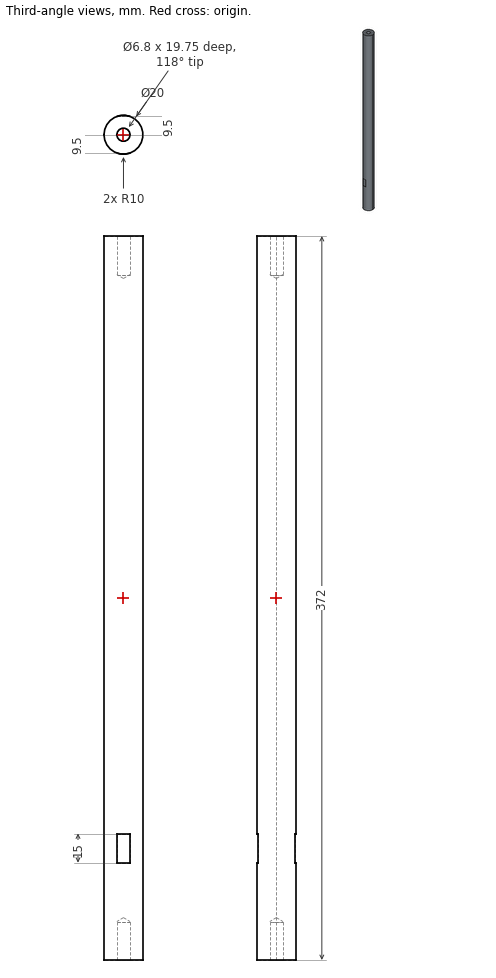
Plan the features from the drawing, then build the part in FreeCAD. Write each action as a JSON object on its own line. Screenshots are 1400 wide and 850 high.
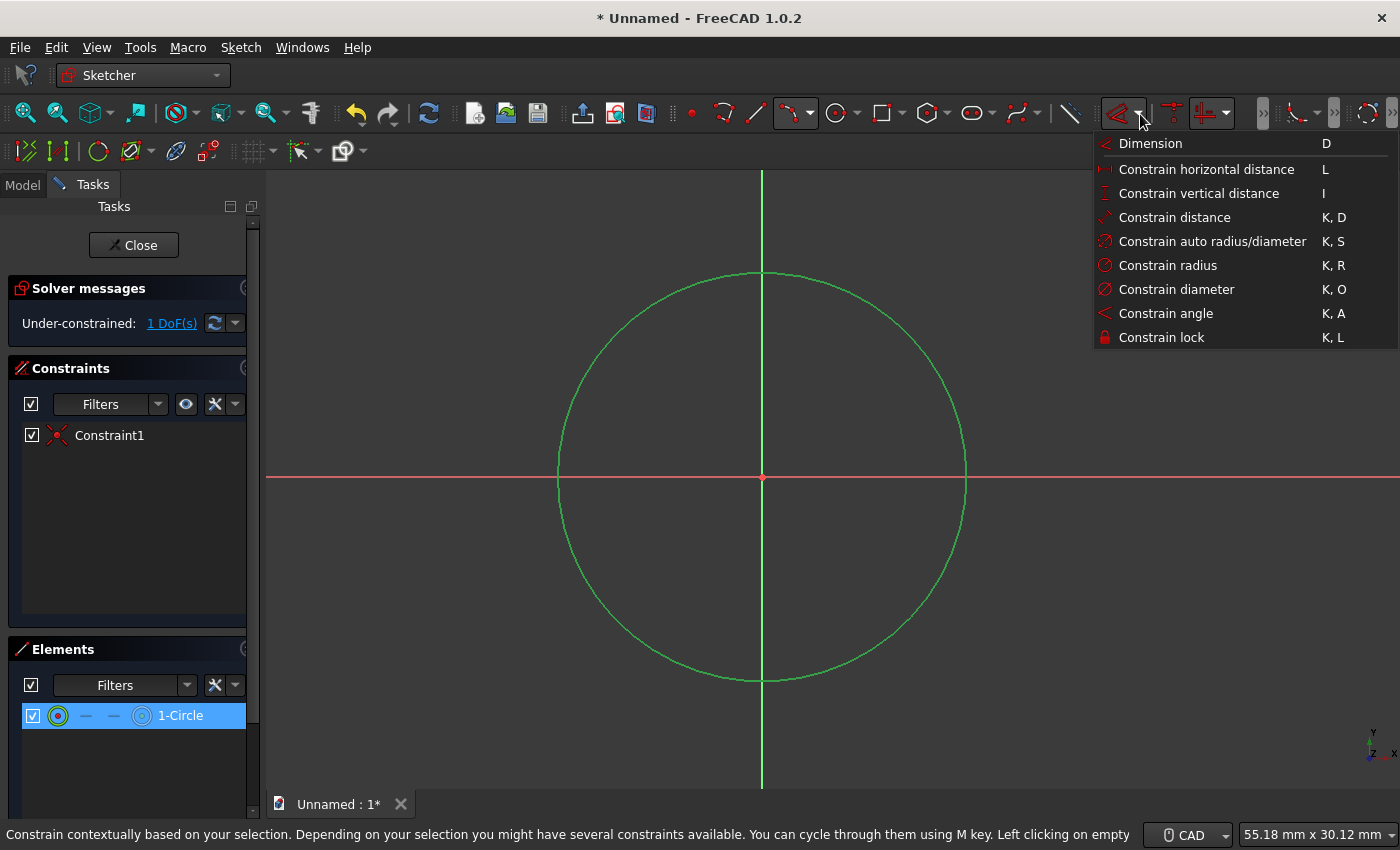
{"action": "left_click", "coordinate": [1246, 289]}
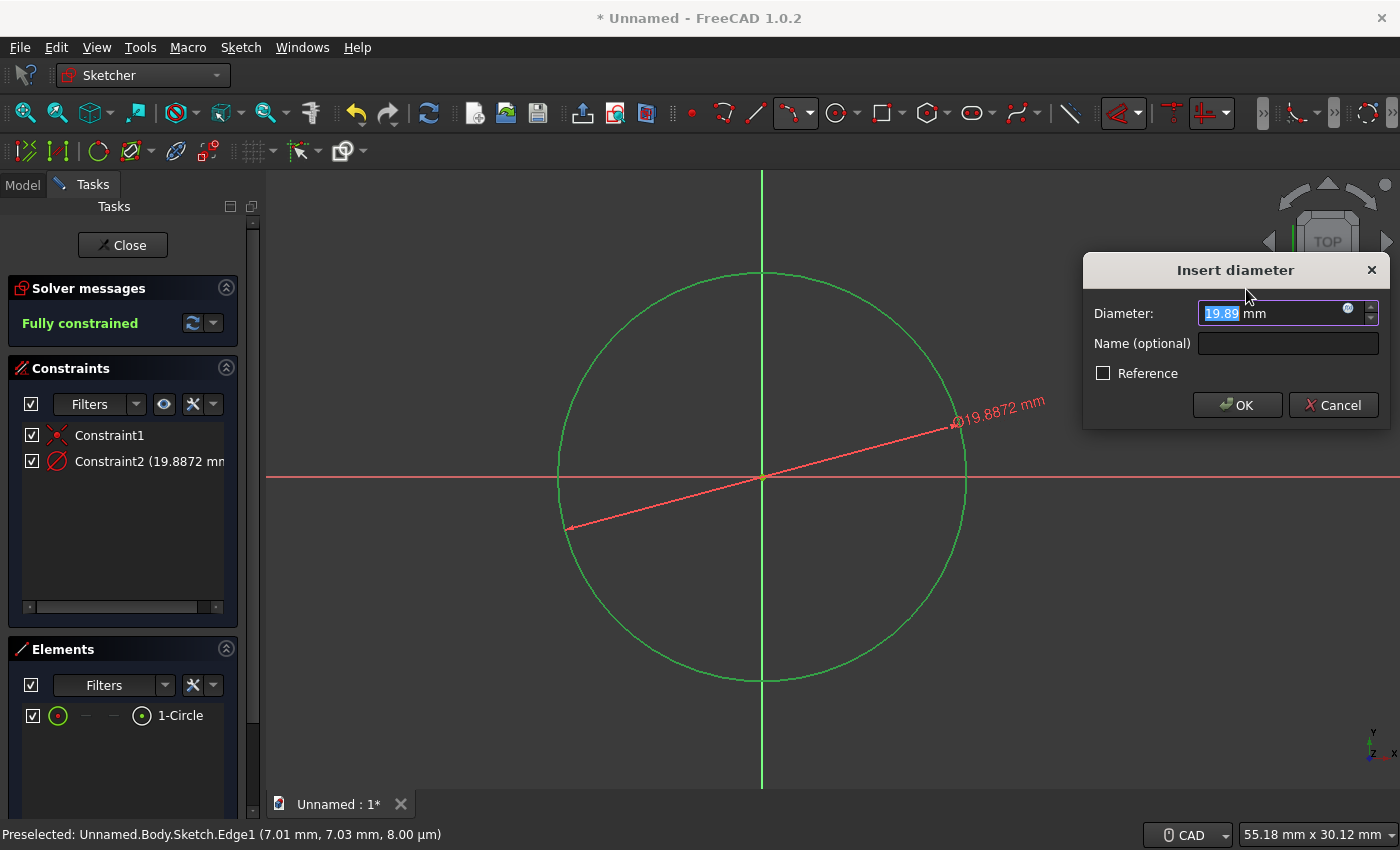
{"action": "type", "text": "20"}
{"action": "key", "text": "Return"}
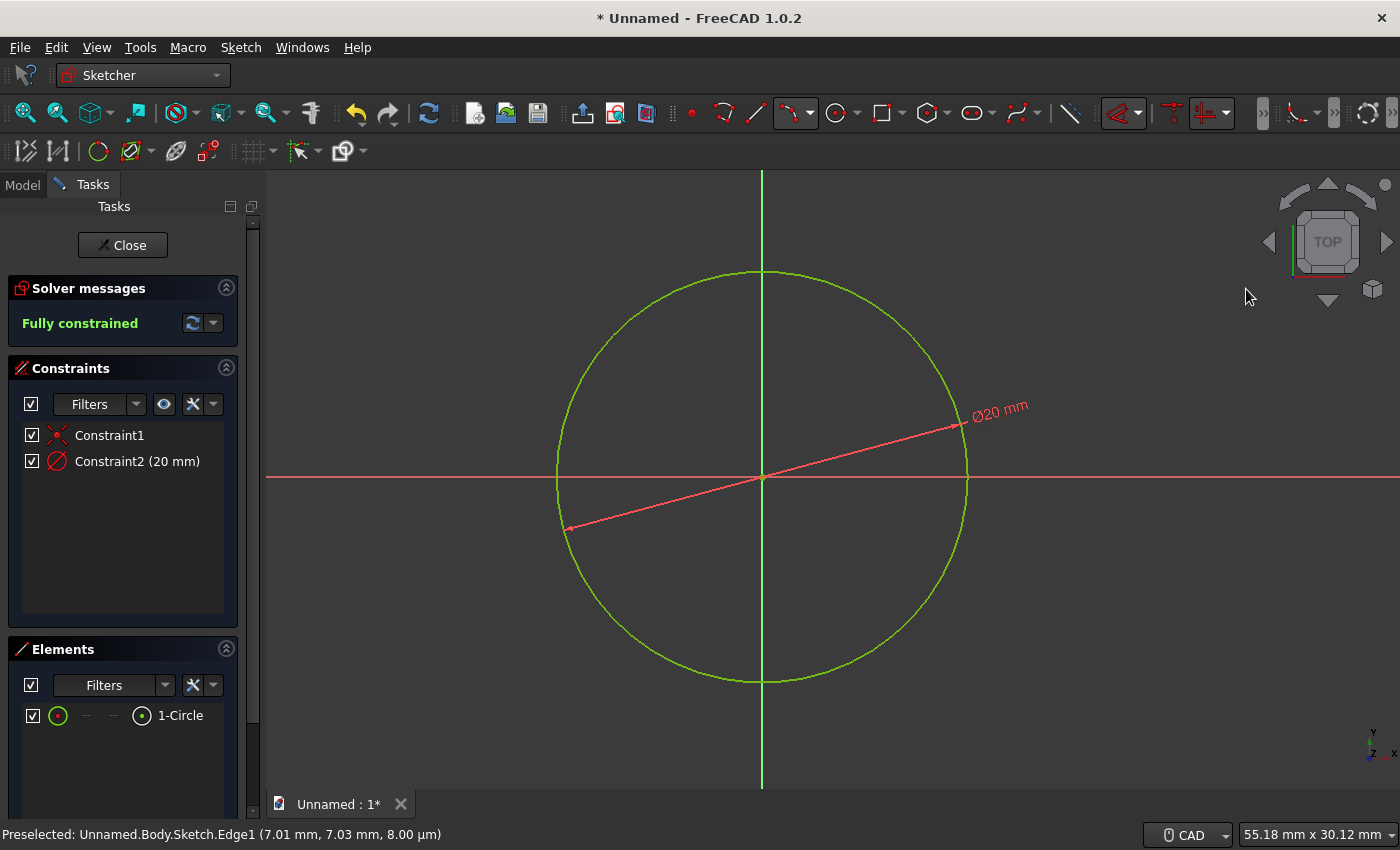
{"action": "left_click", "coordinate": [123, 245]}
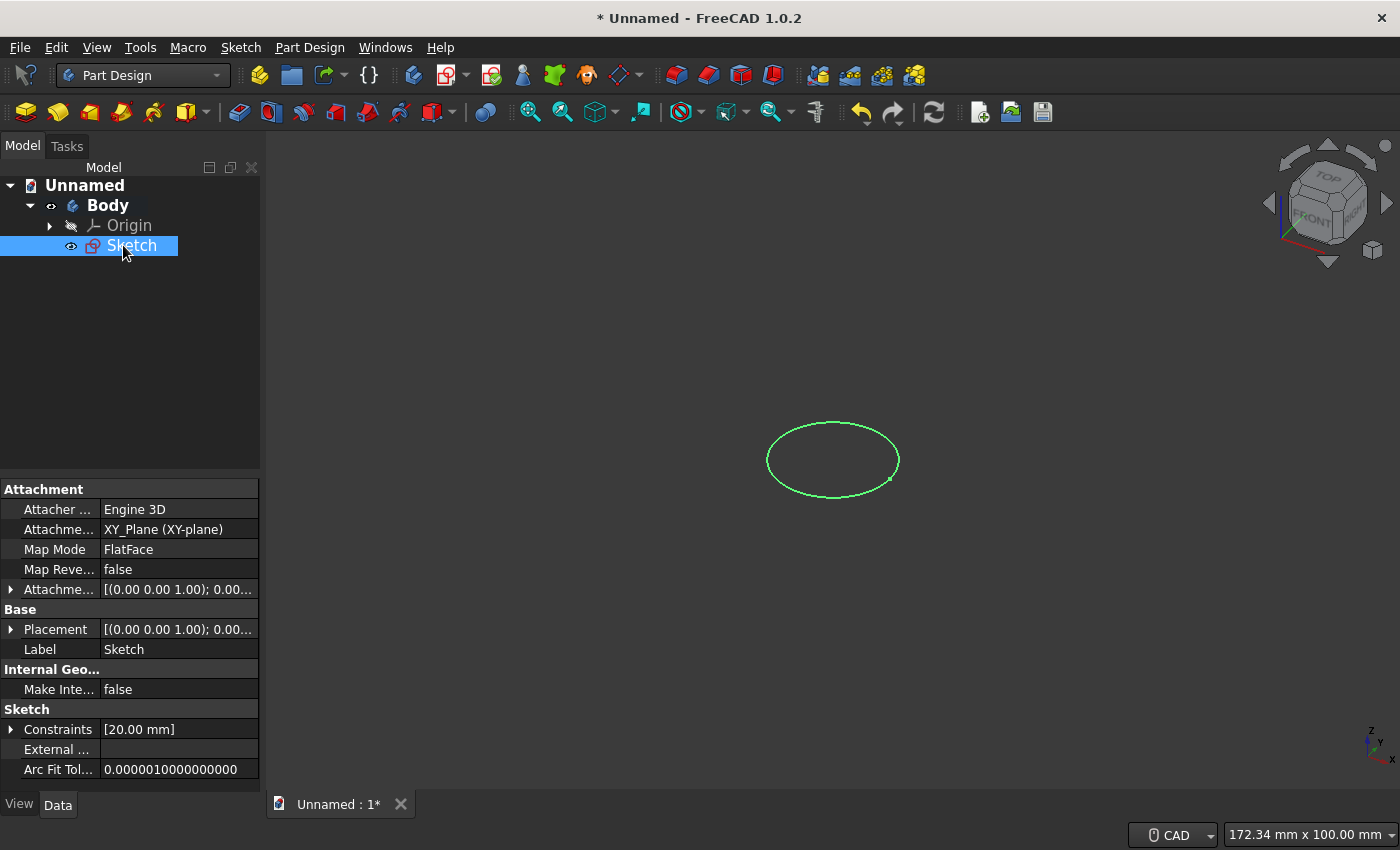
{"action": "left_click", "coordinate": [26, 112]}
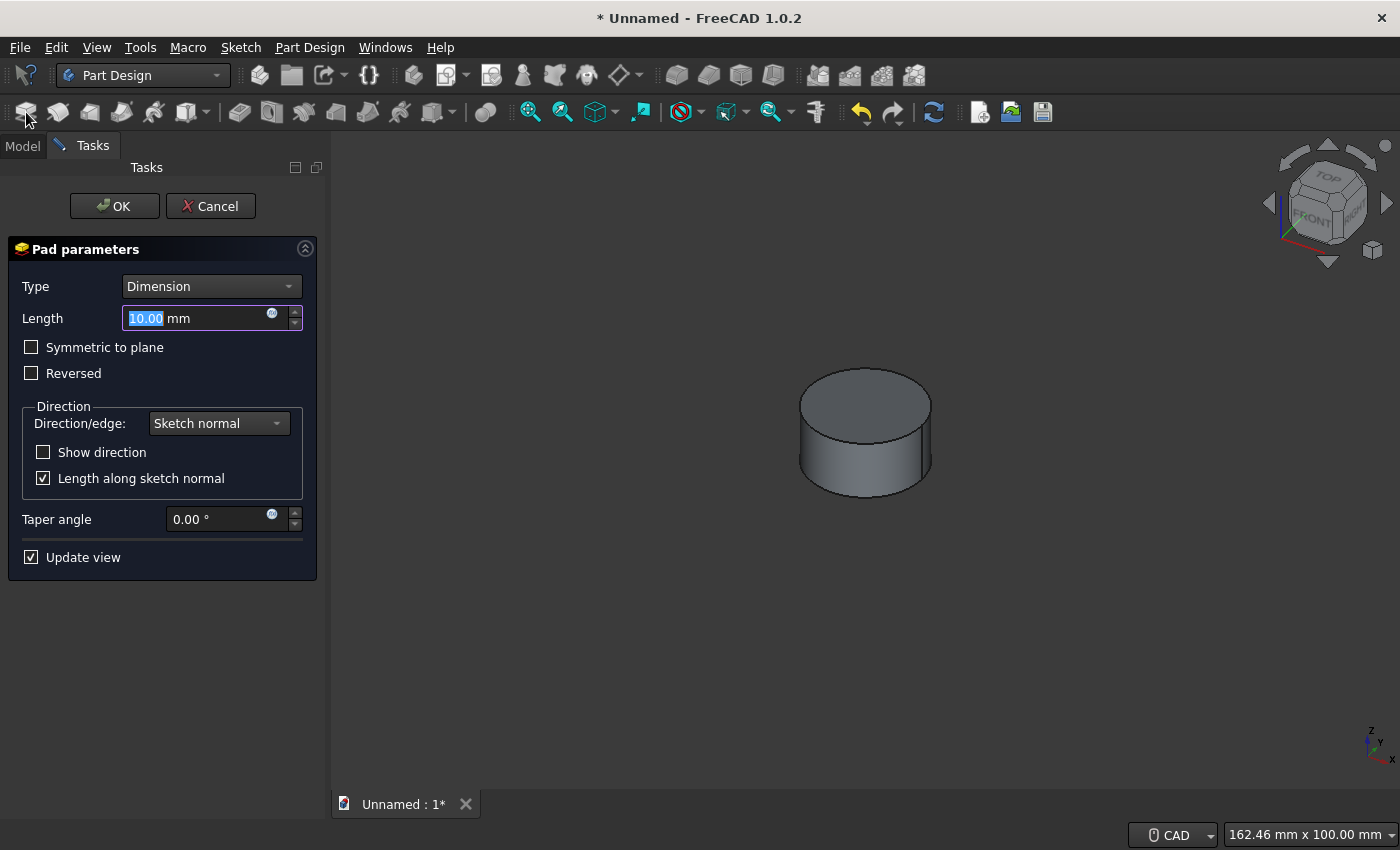
{"action": "type", "text": "372"}
{"action": "key", "text": "Tab"}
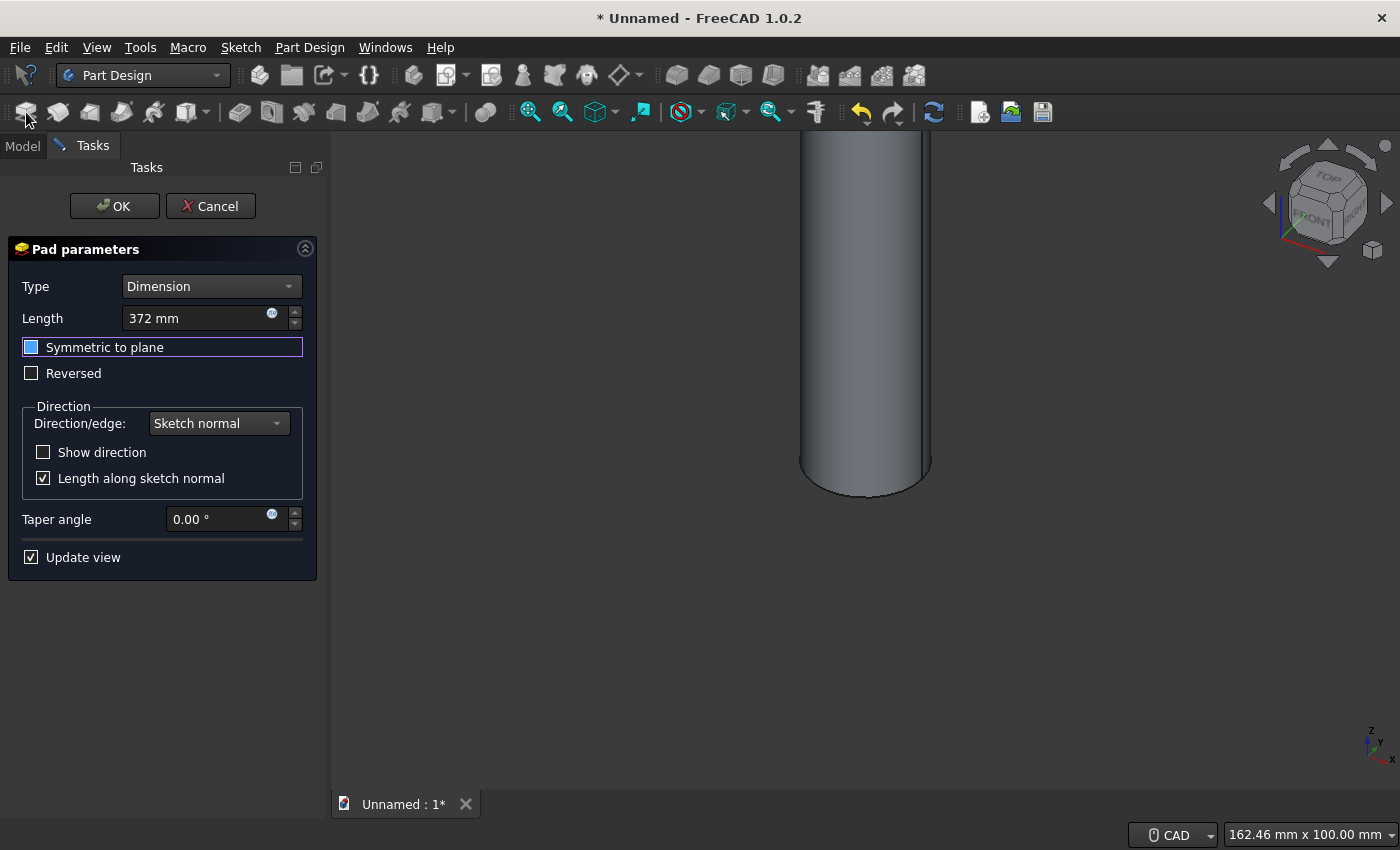
{"action": "left_click", "coordinate": [30, 347]}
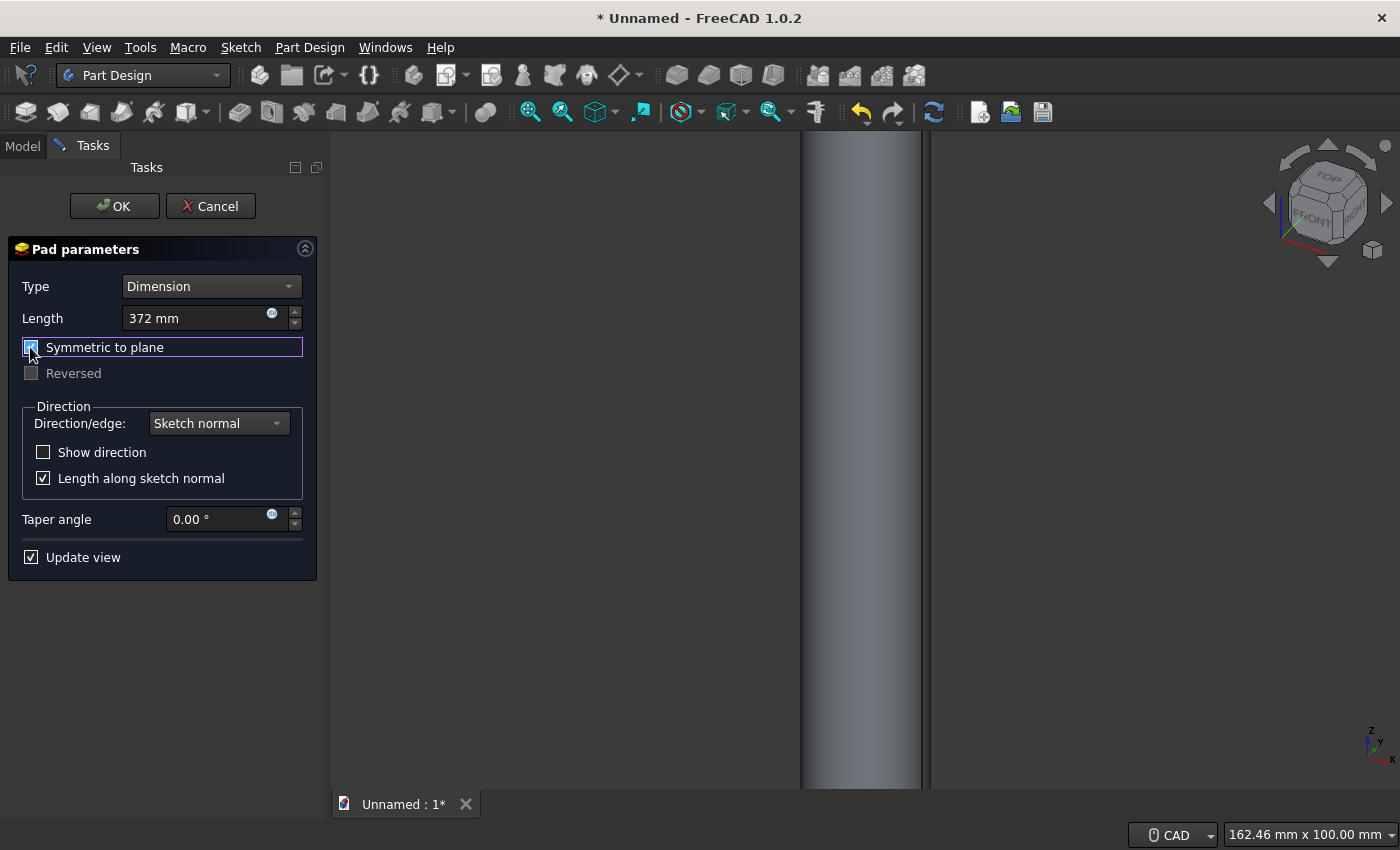
{"action": "left_click", "coordinate": [115, 206]}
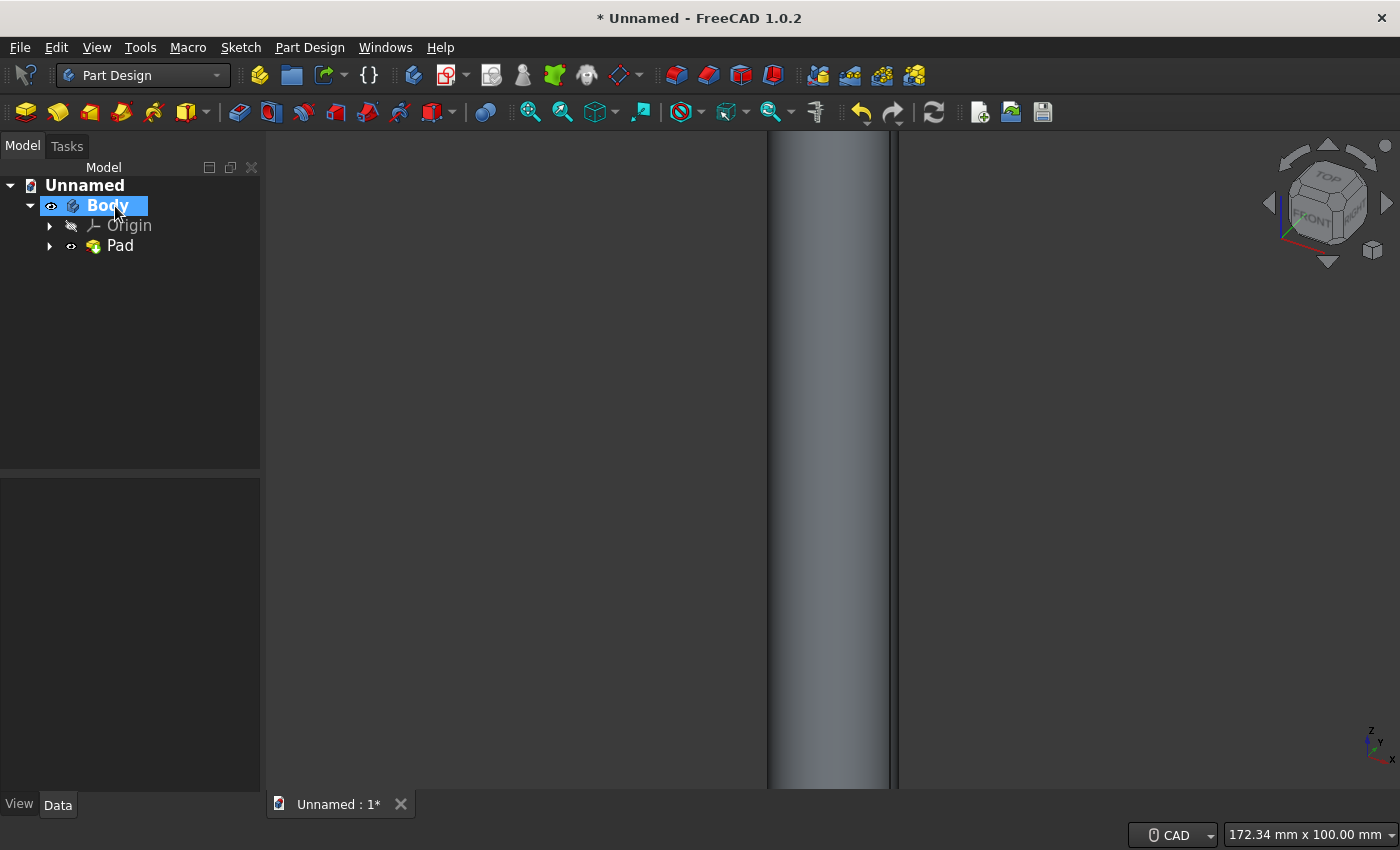
{"action": "key", "text": "v f"}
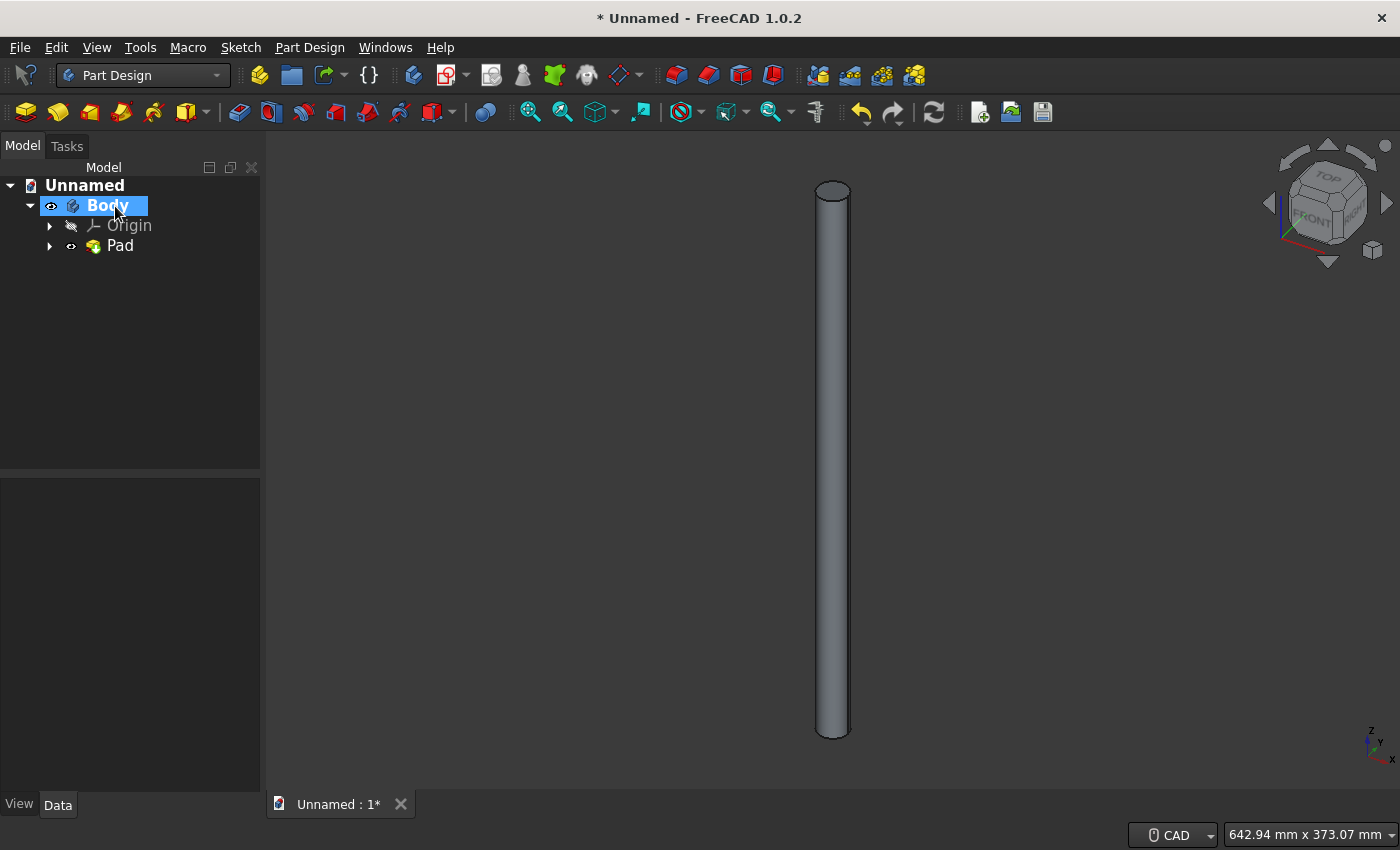
{"action": "left_click", "coordinate": [50, 226]}